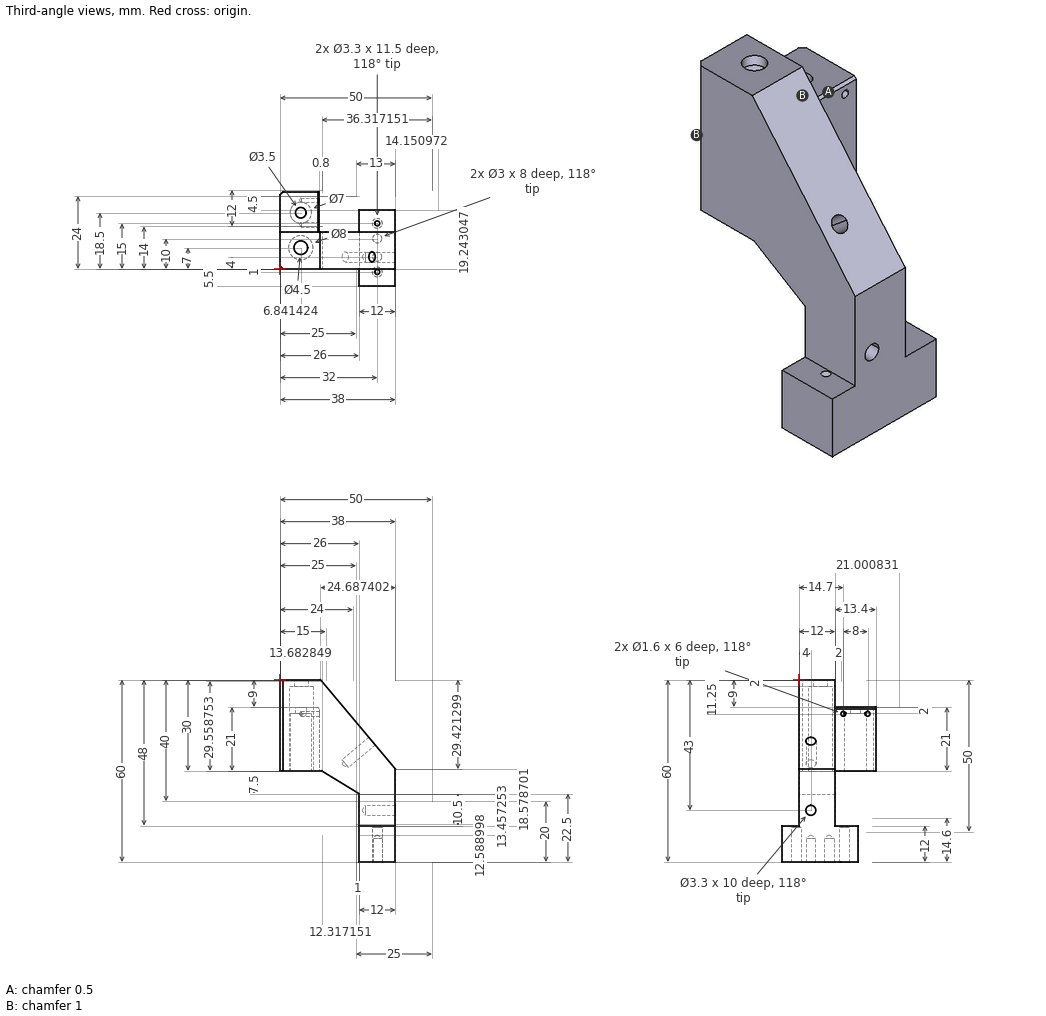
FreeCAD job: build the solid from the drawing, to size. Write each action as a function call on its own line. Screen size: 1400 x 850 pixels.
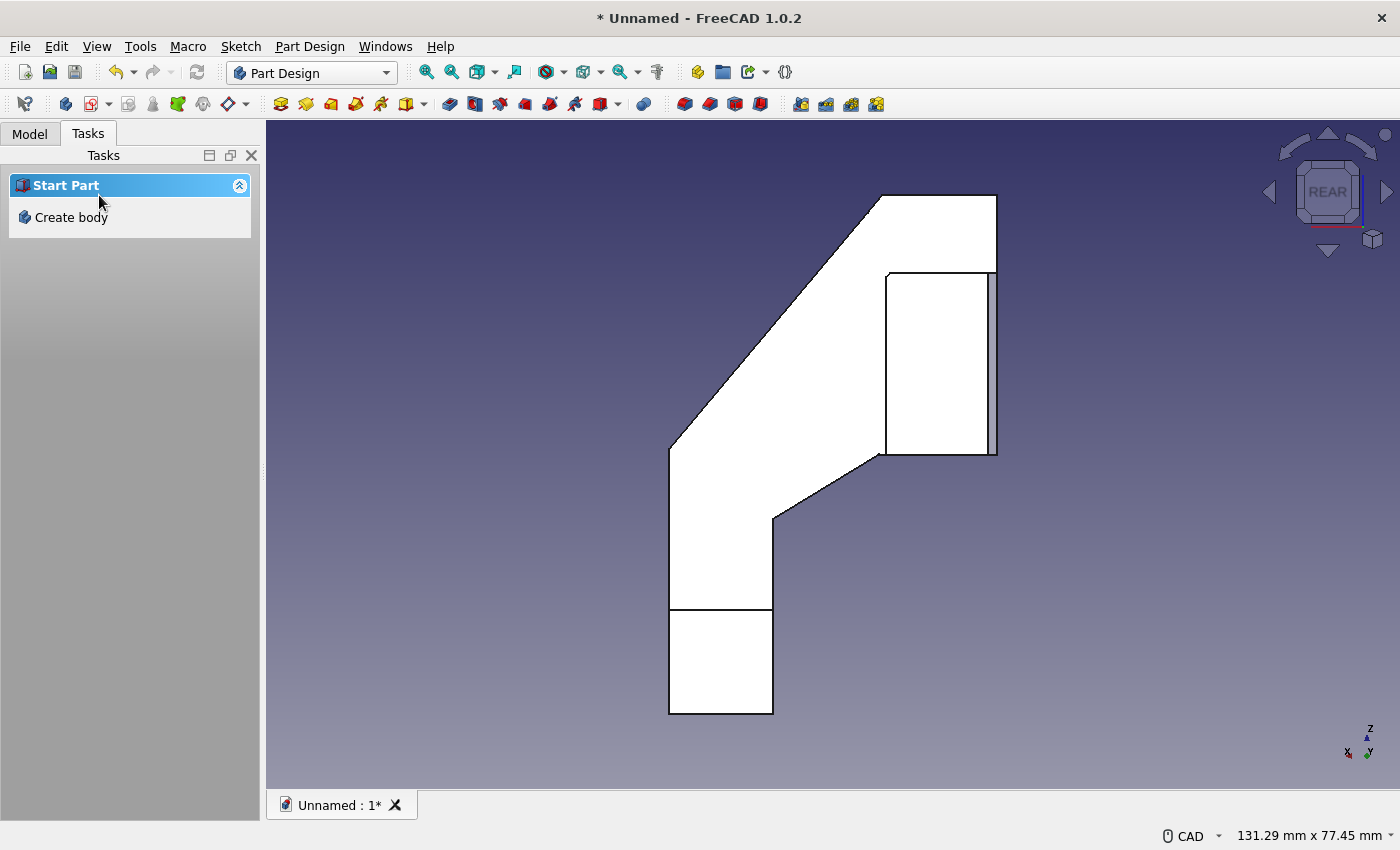
key(0)